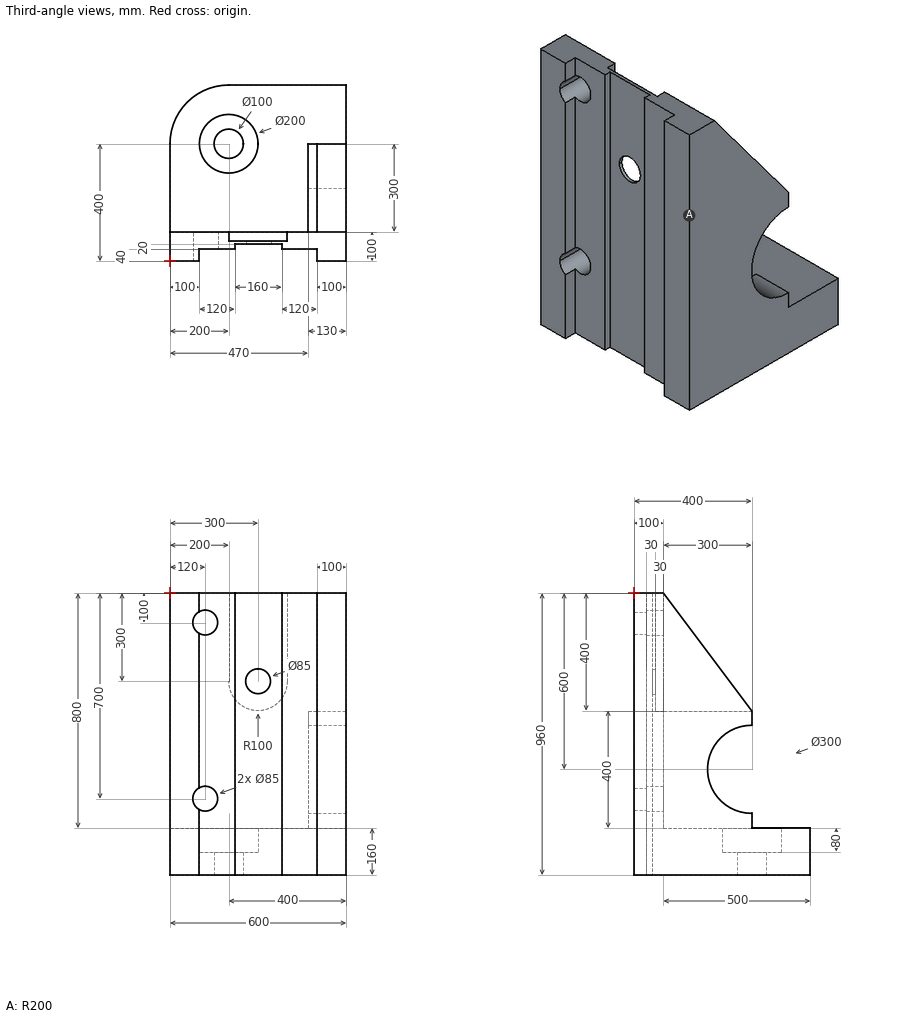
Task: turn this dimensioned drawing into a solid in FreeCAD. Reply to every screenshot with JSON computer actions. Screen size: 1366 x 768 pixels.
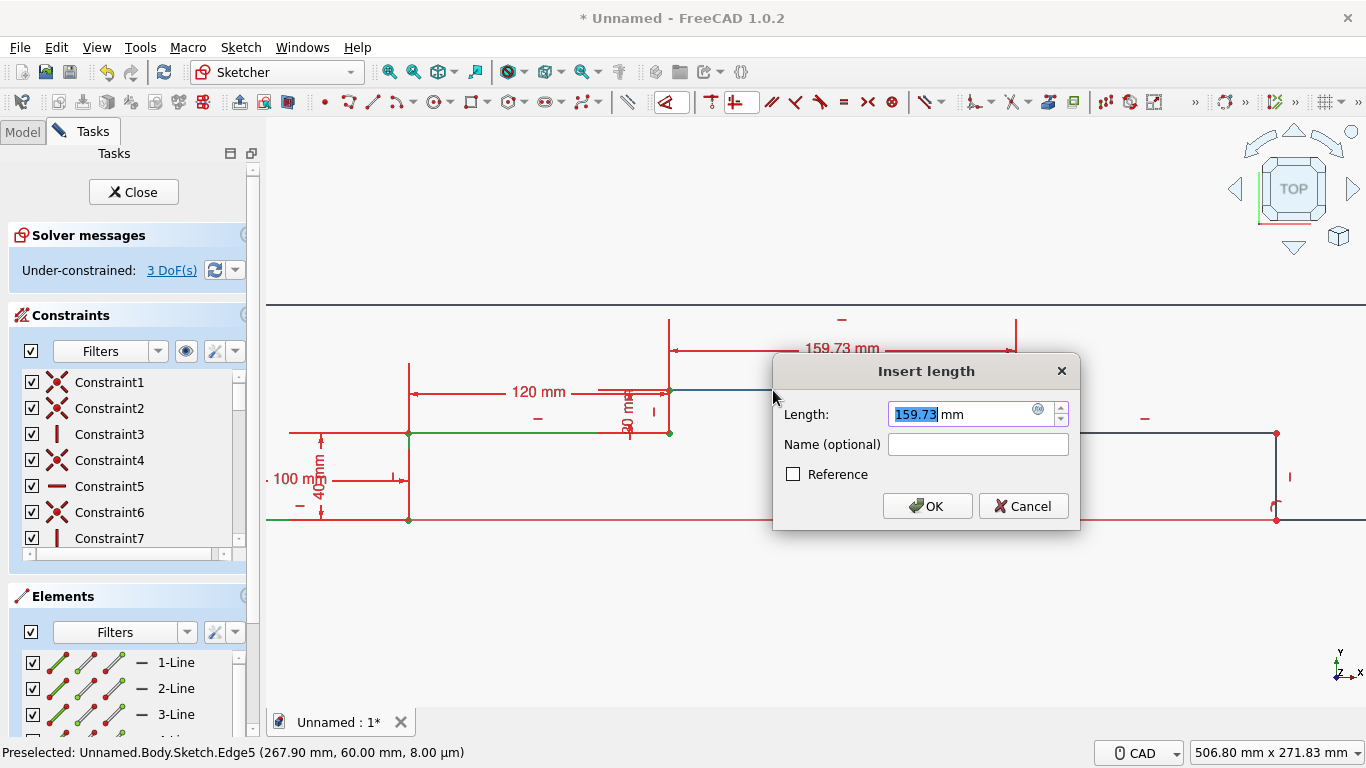
{"action": "type", "text": "160"}
{"action": "key", "text": "Return"}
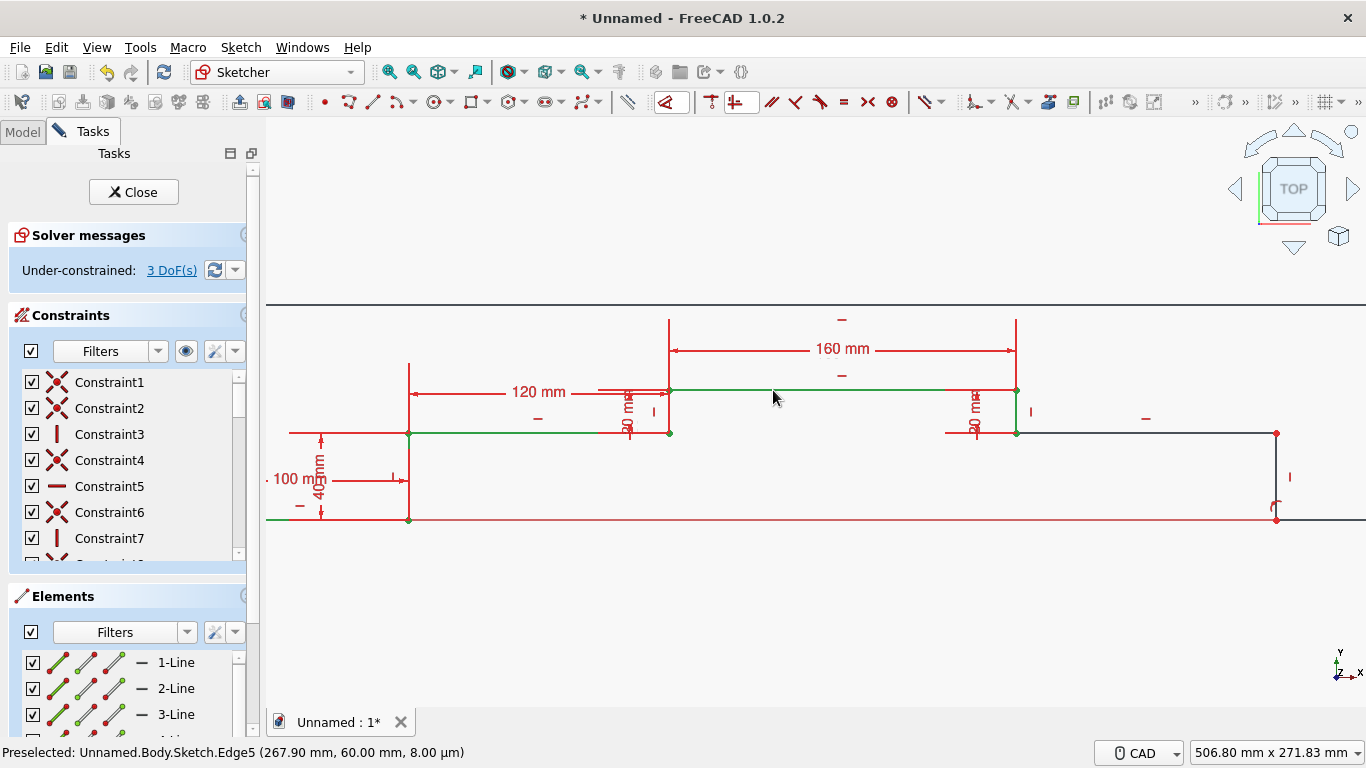
{"action": "left_click", "coordinate": [1094, 433]}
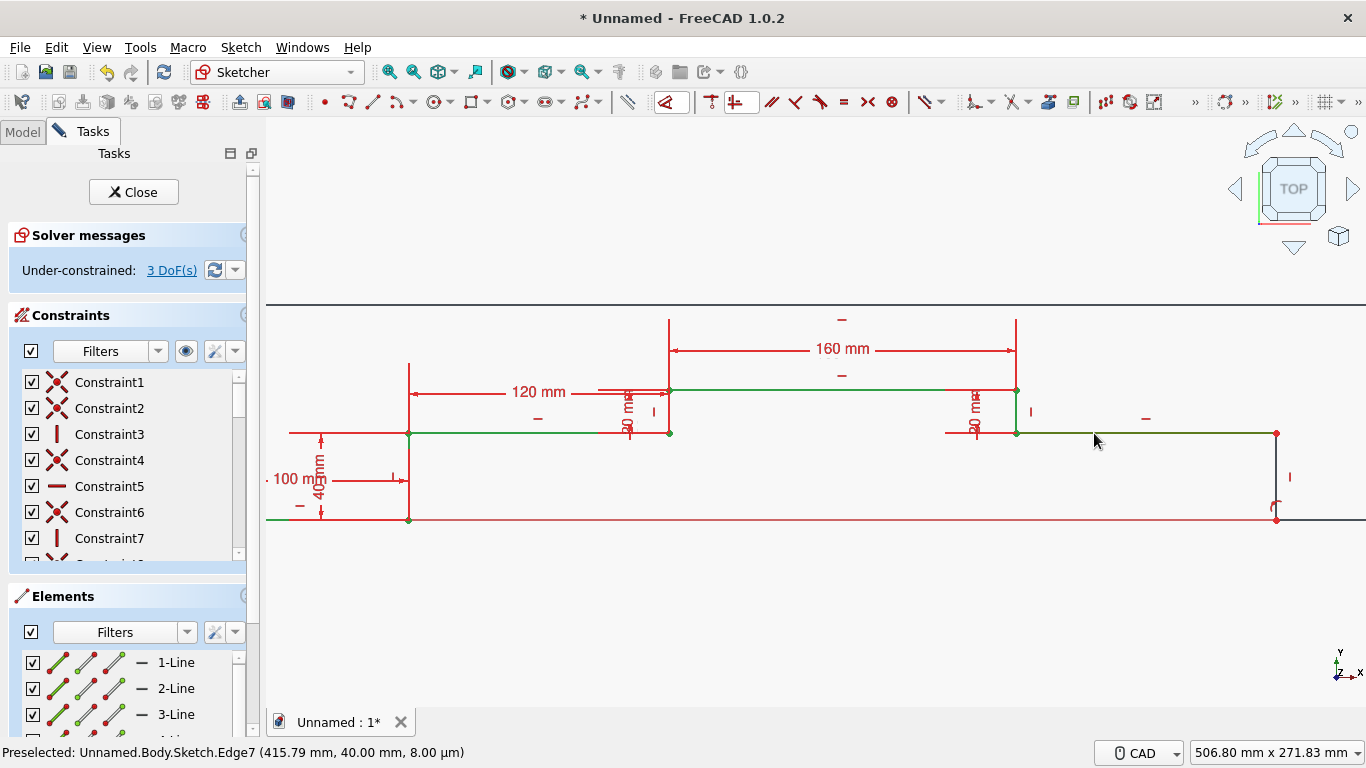
{"action": "key", "text": "l"}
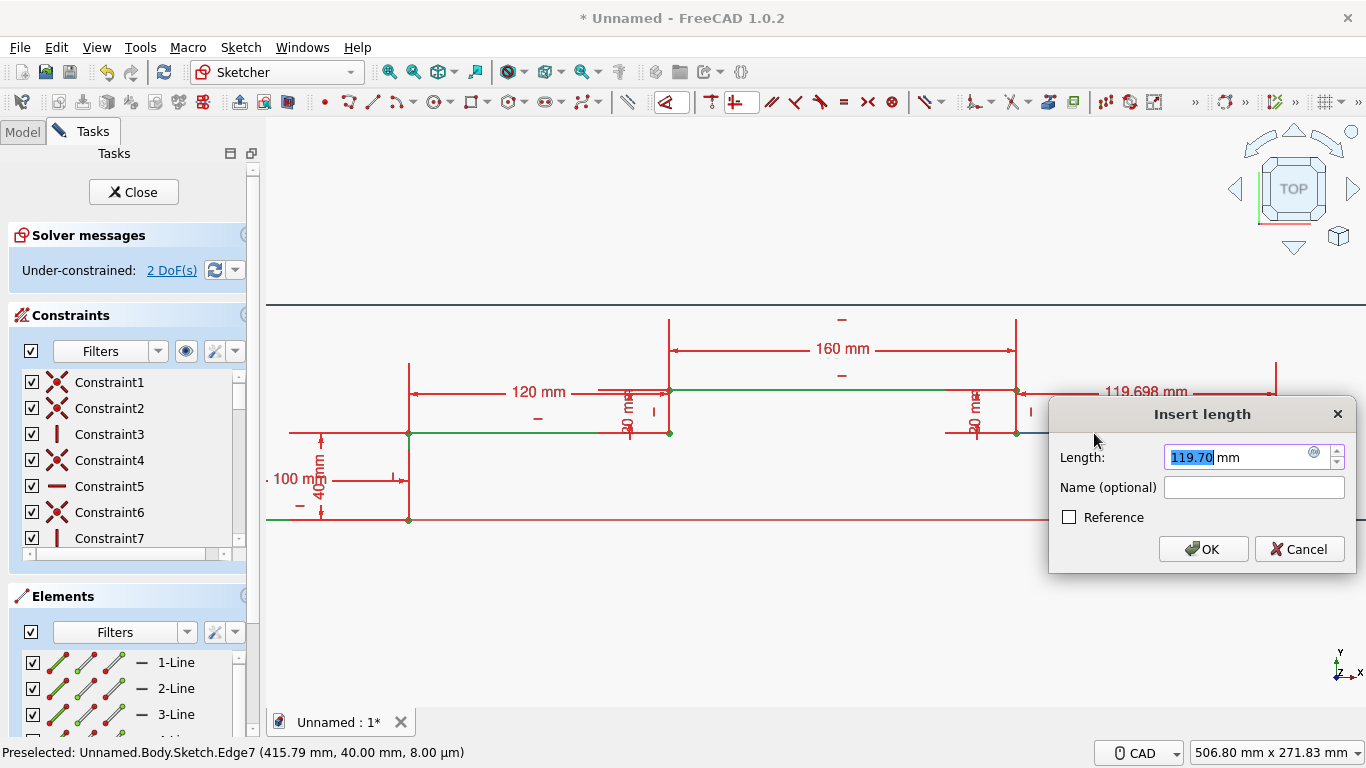
{"action": "type", "text": "120"}
{"action": "key", "text": "Return"}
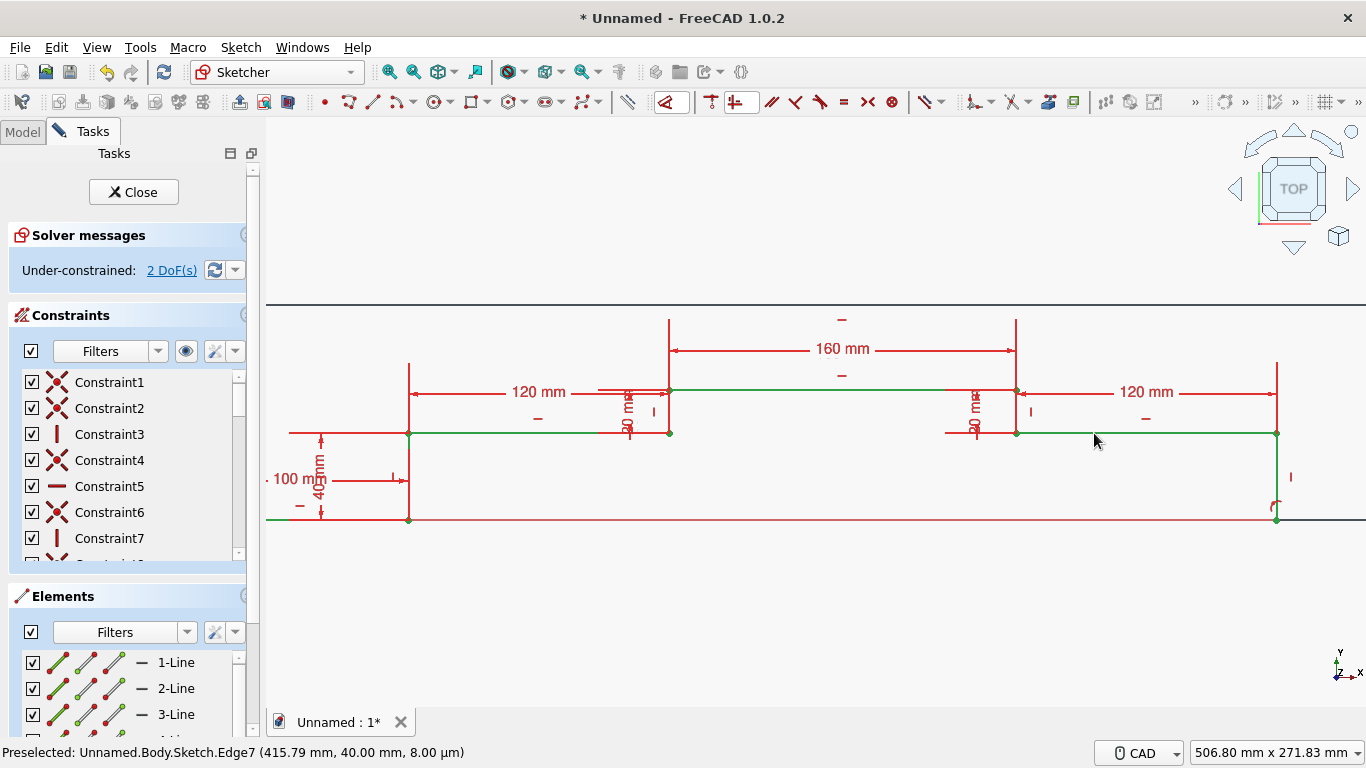
{"action": "scroll", "coordinate": [670, 412], "scroll_direction": "down", "scroll_amount": 4}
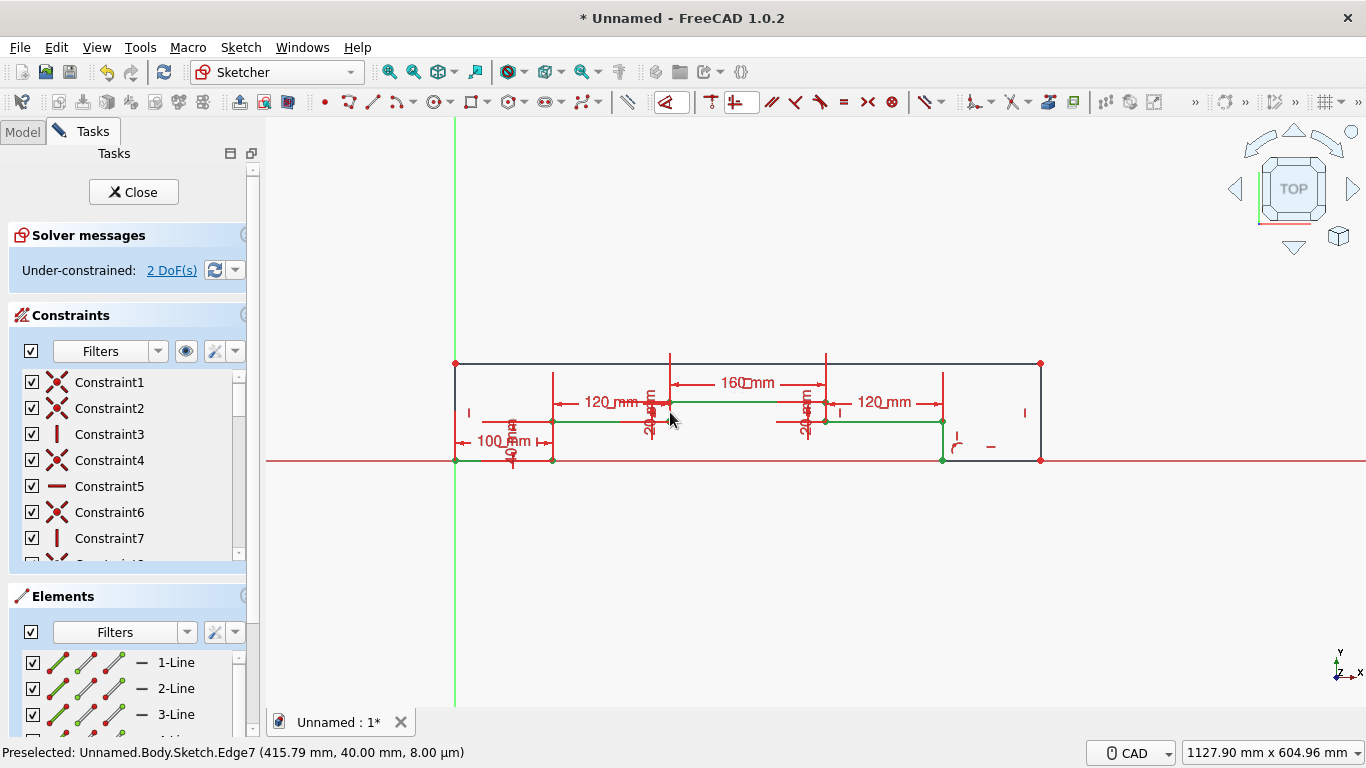
{"action": "left_click", "coordinate": [972, 461]}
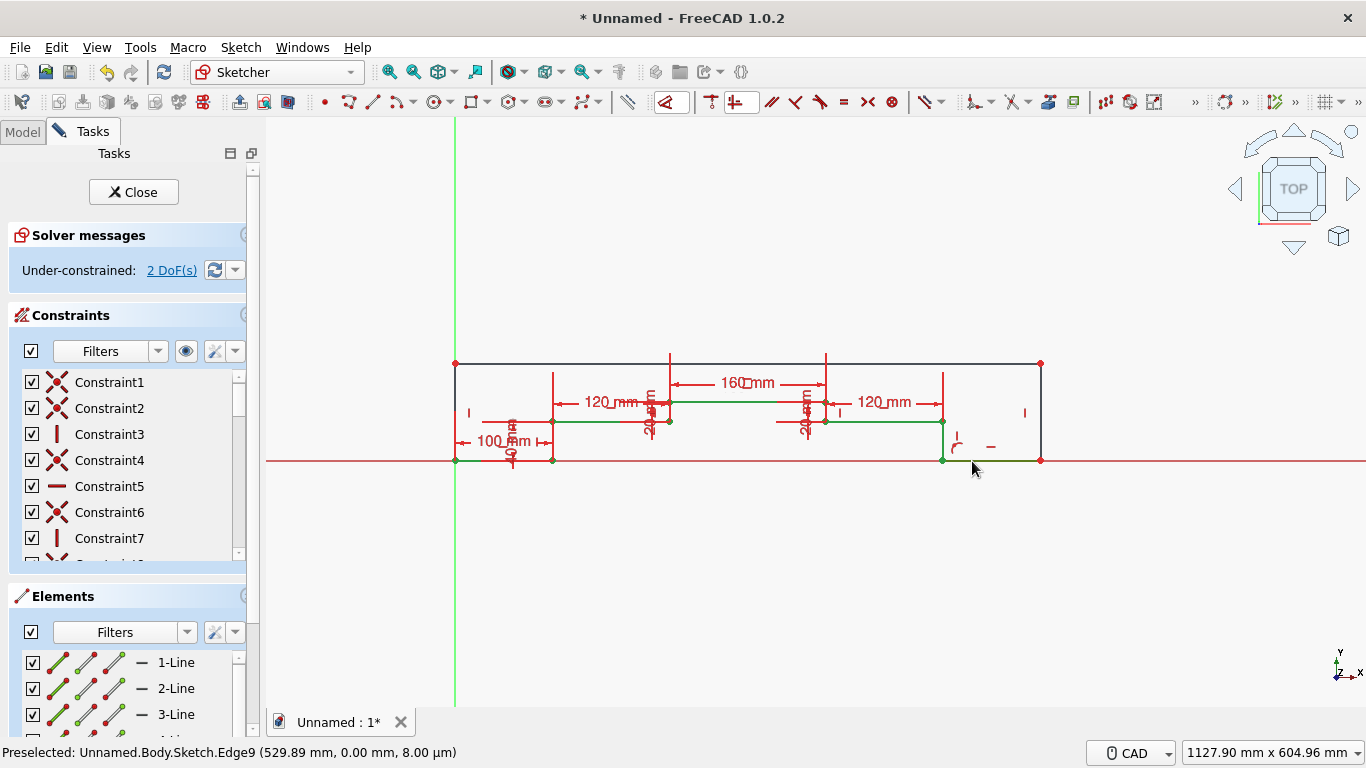
{"action": "left_click", "coordinate": [684, 102]}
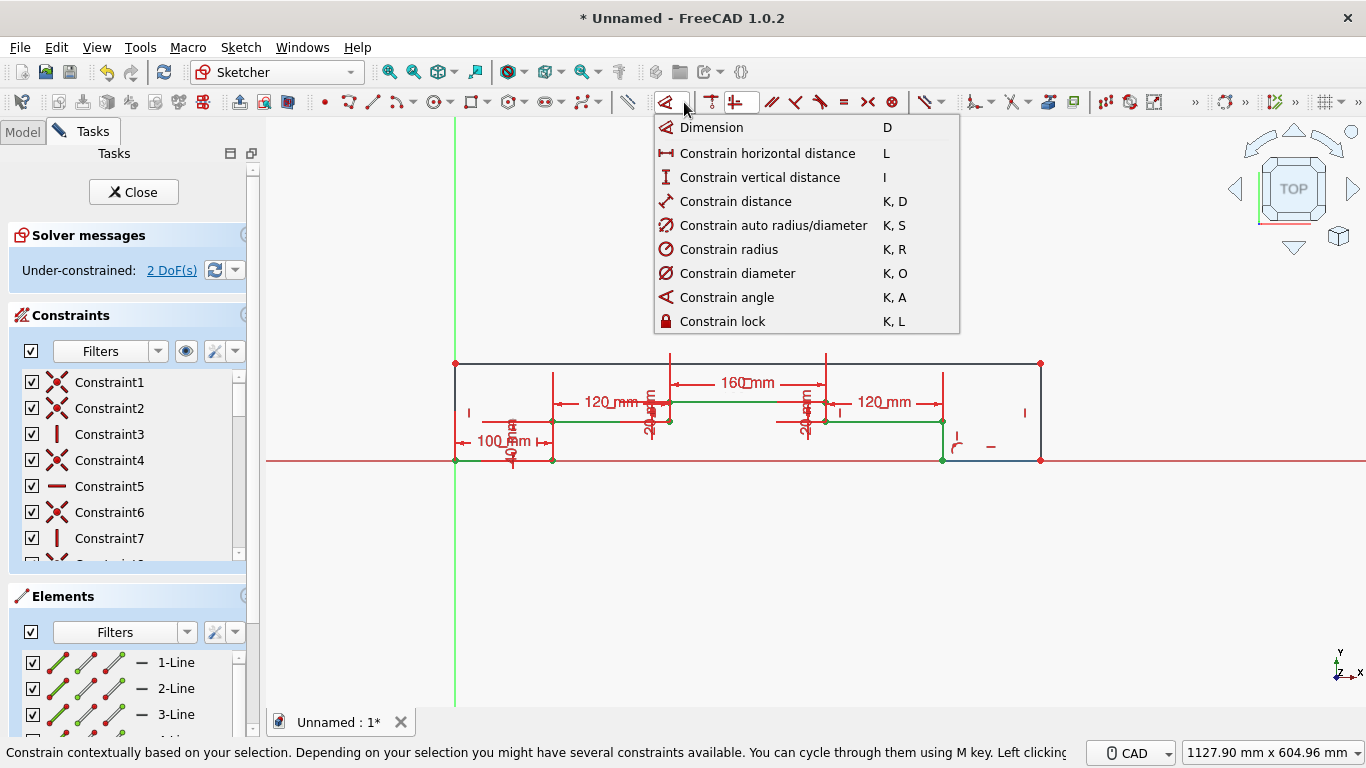
{"action": "left_click", "coordinate": [807, 153]}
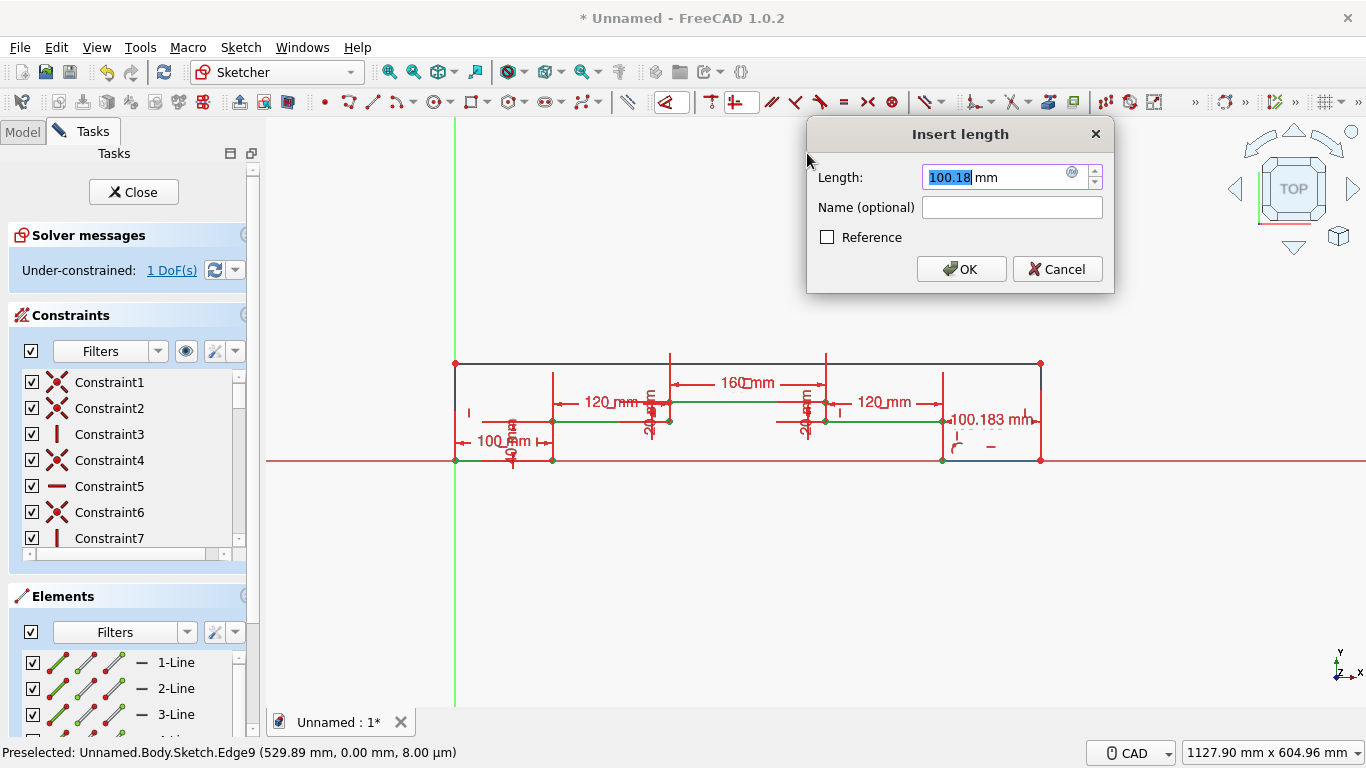
{"action": "type", "text": "100"}
{"action": "key", "text": "Return"}